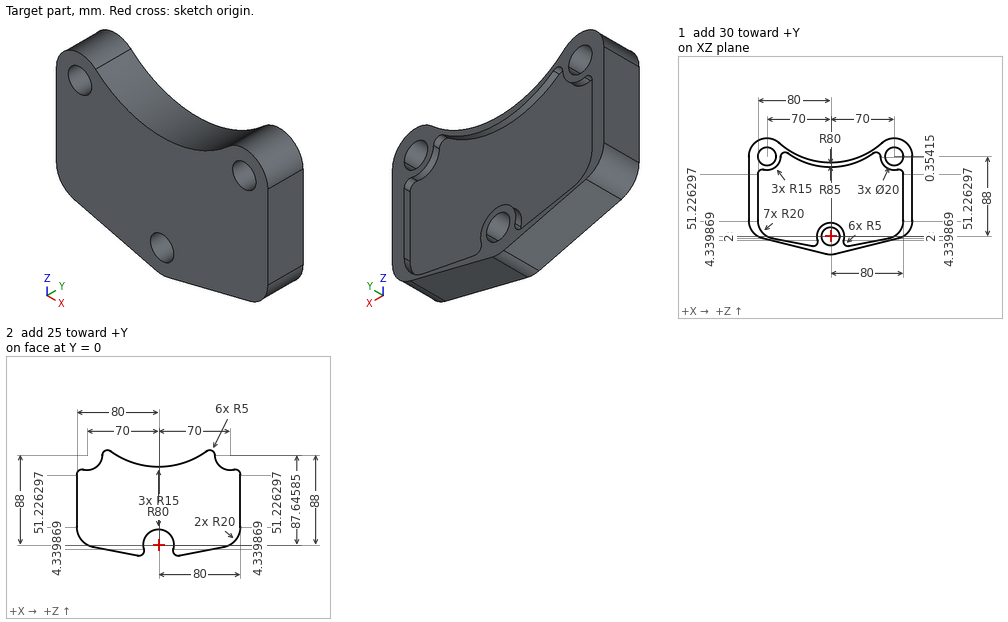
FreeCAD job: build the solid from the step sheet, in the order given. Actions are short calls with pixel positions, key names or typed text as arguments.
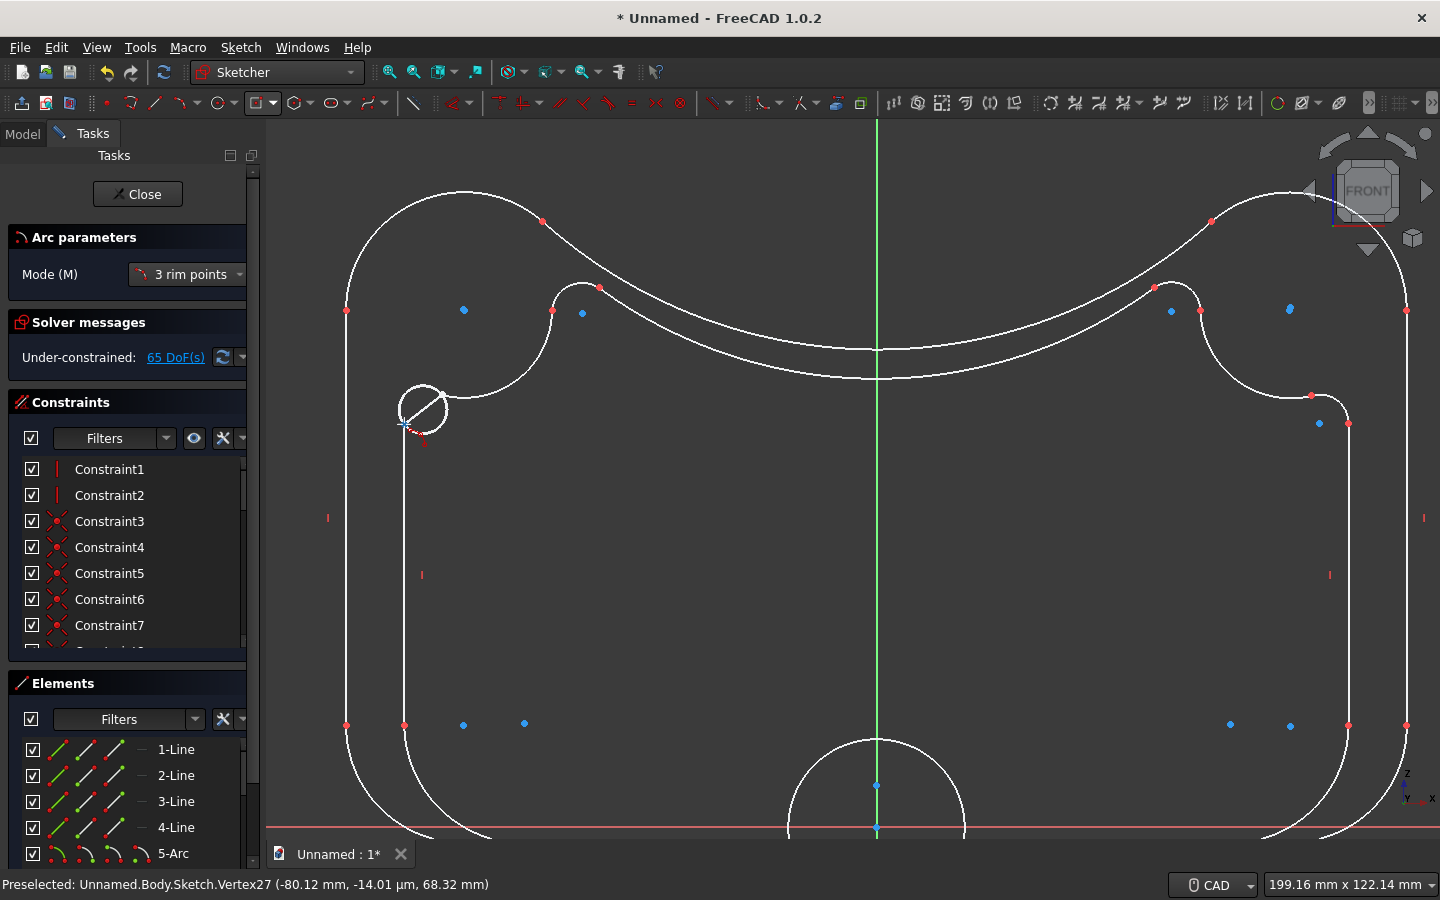
scroll(416, 399, up, 2)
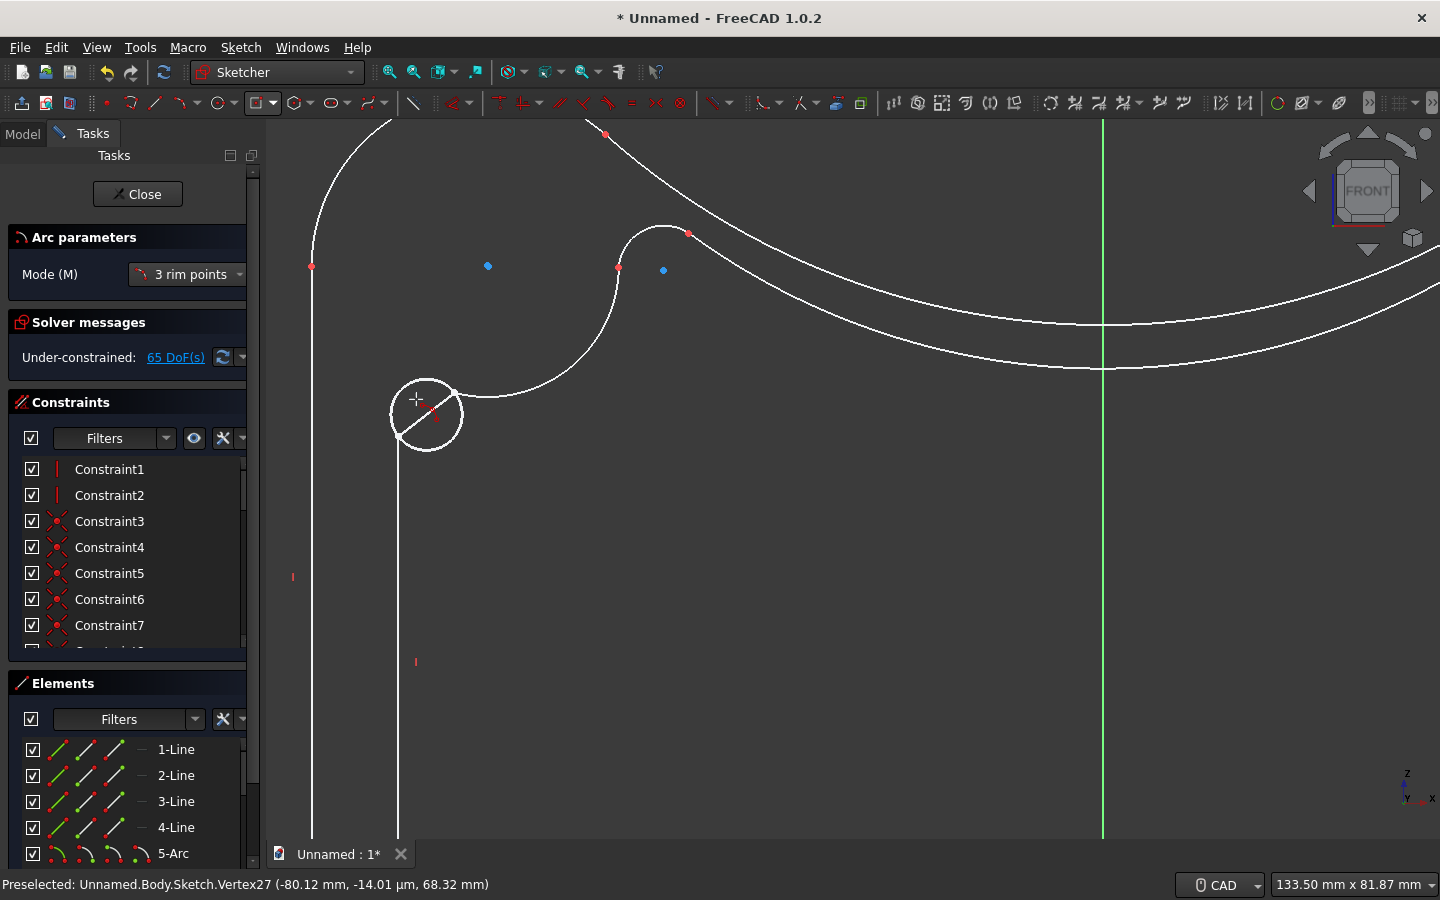
click(417, 399)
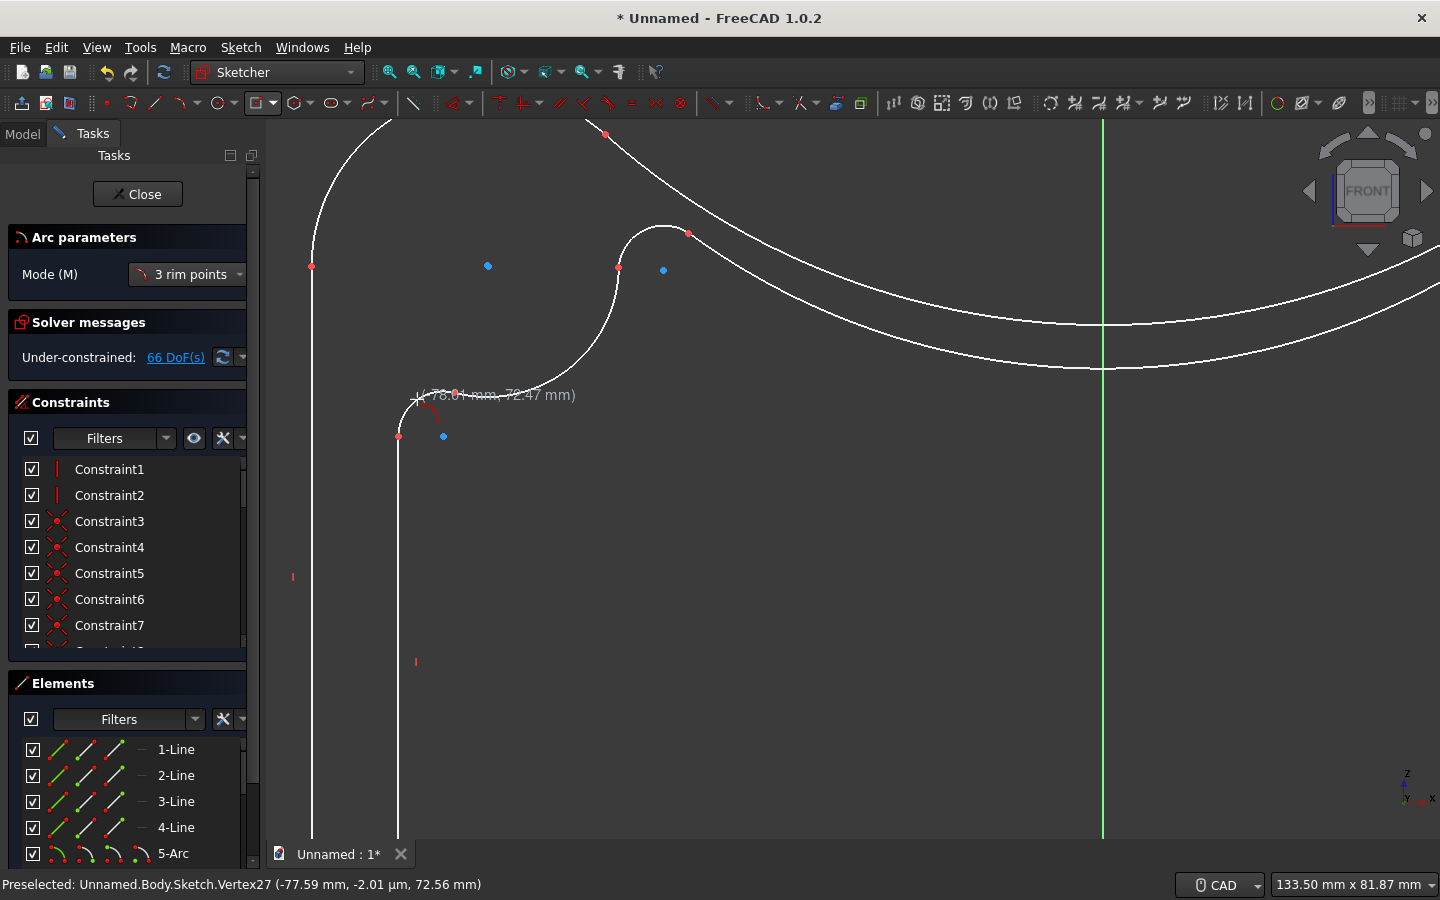
key(g)
key(c)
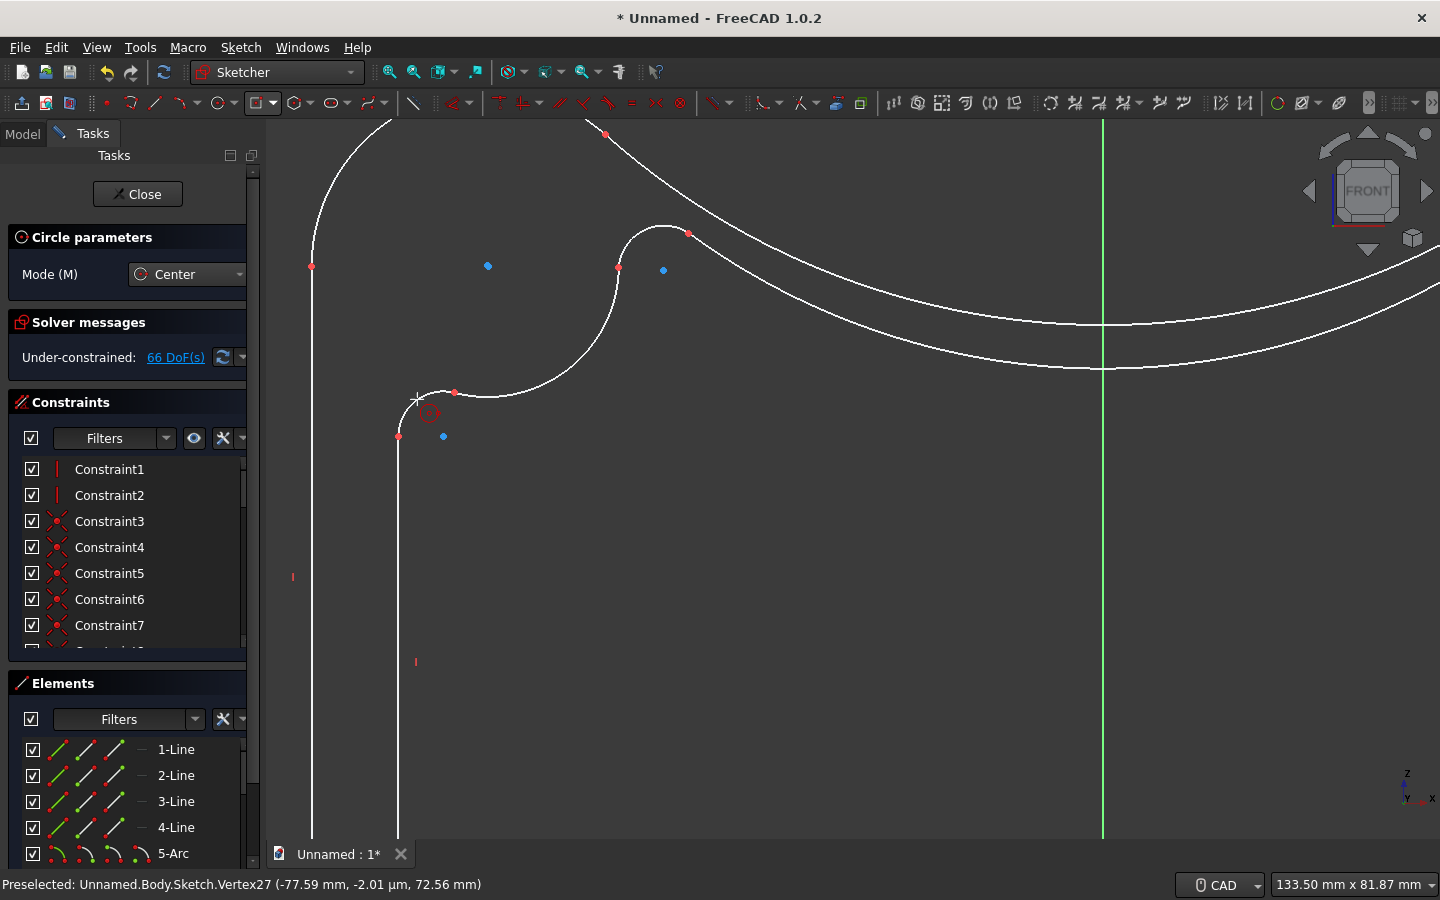
scroll(525, 333, down, 4)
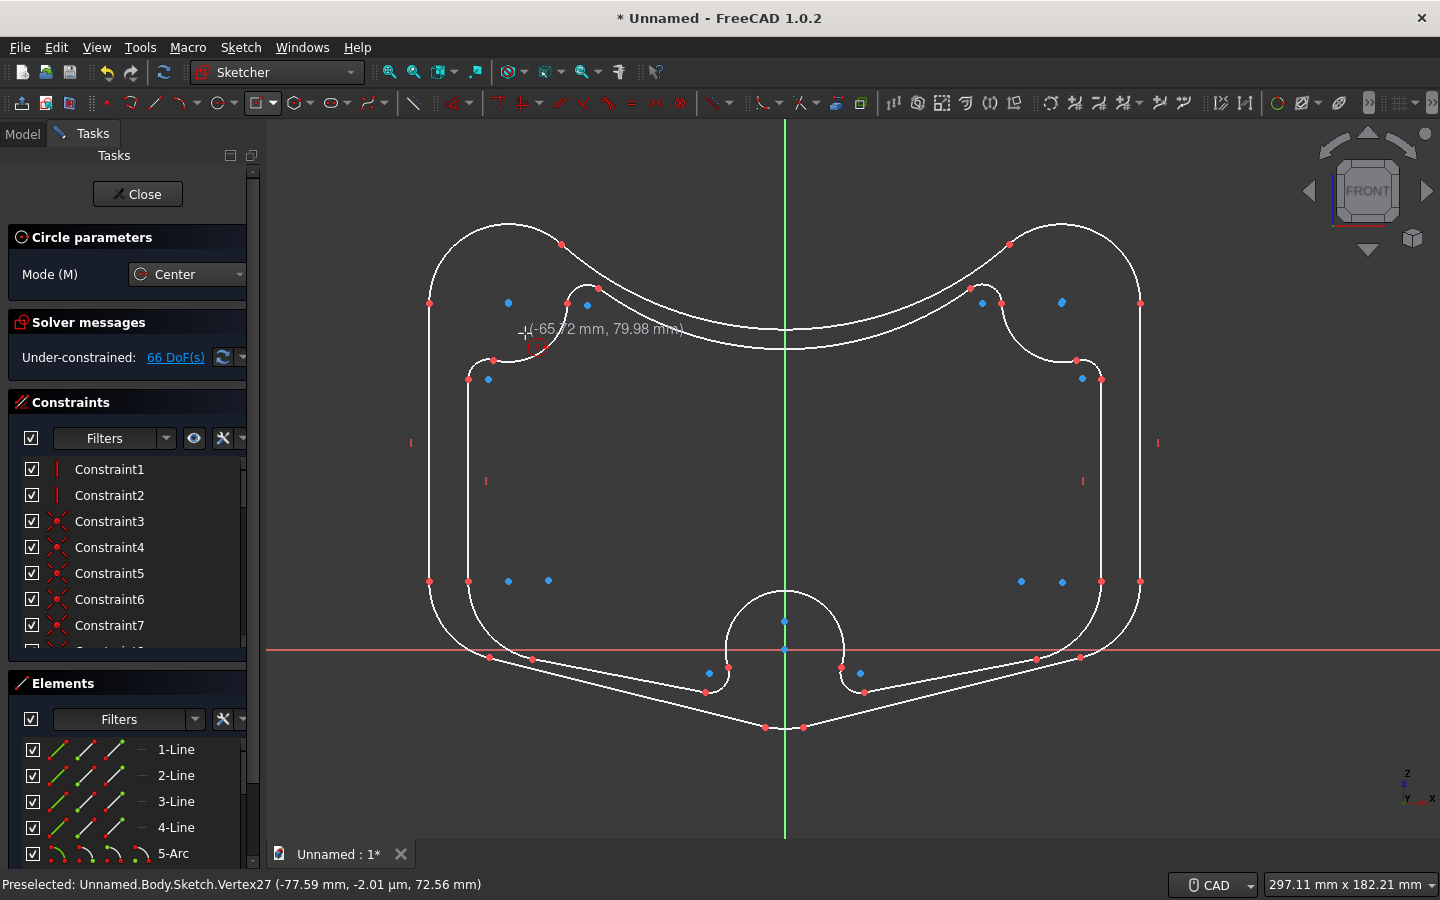
click(1061, 302)
move(1089, 274)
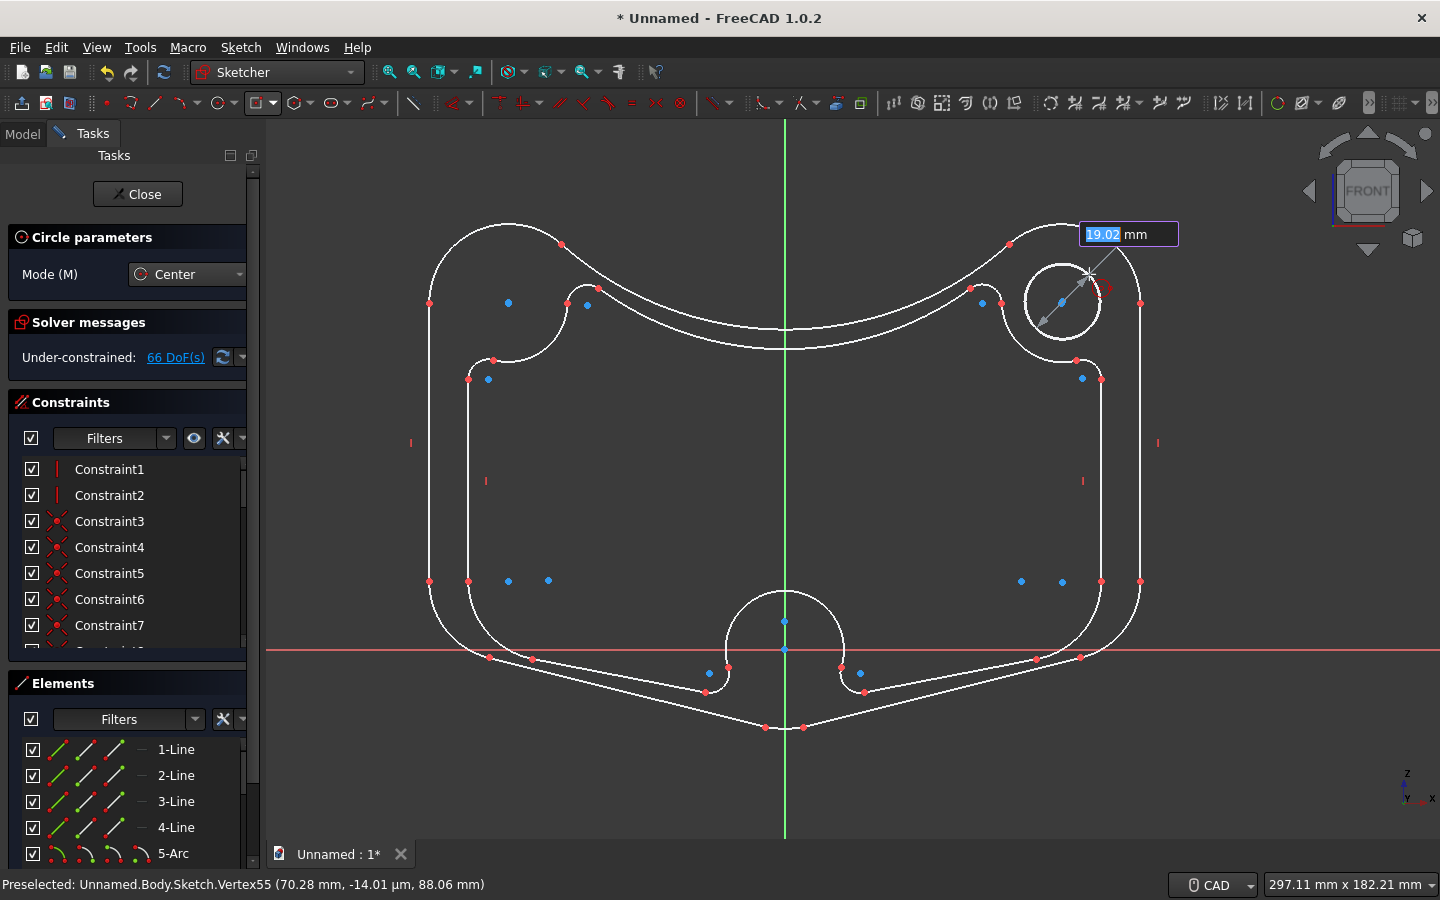
text(20)
key(Return)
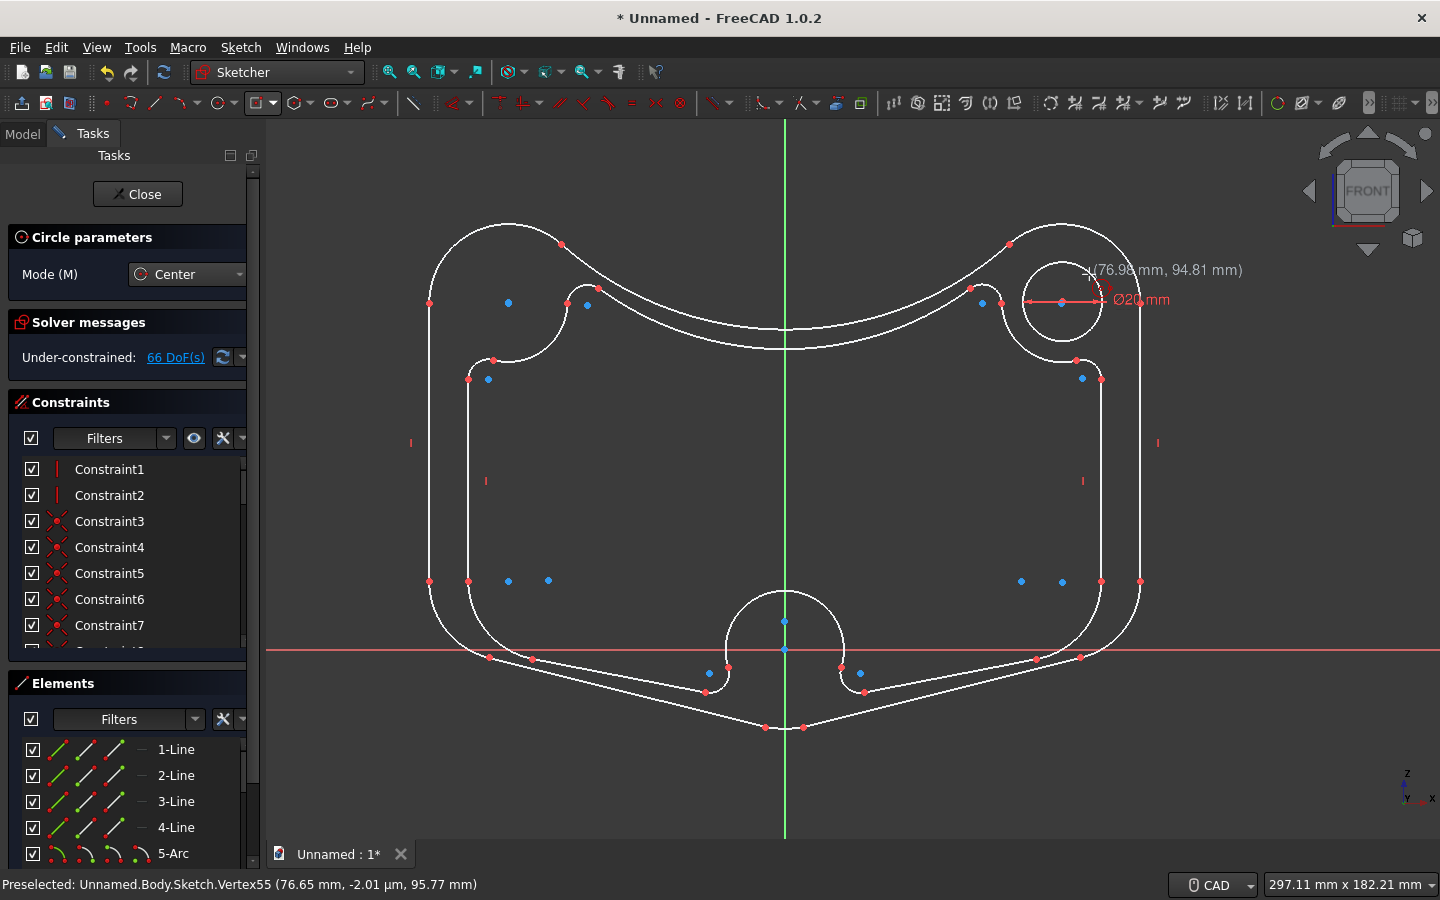
click(508, 302)
move(536, 274)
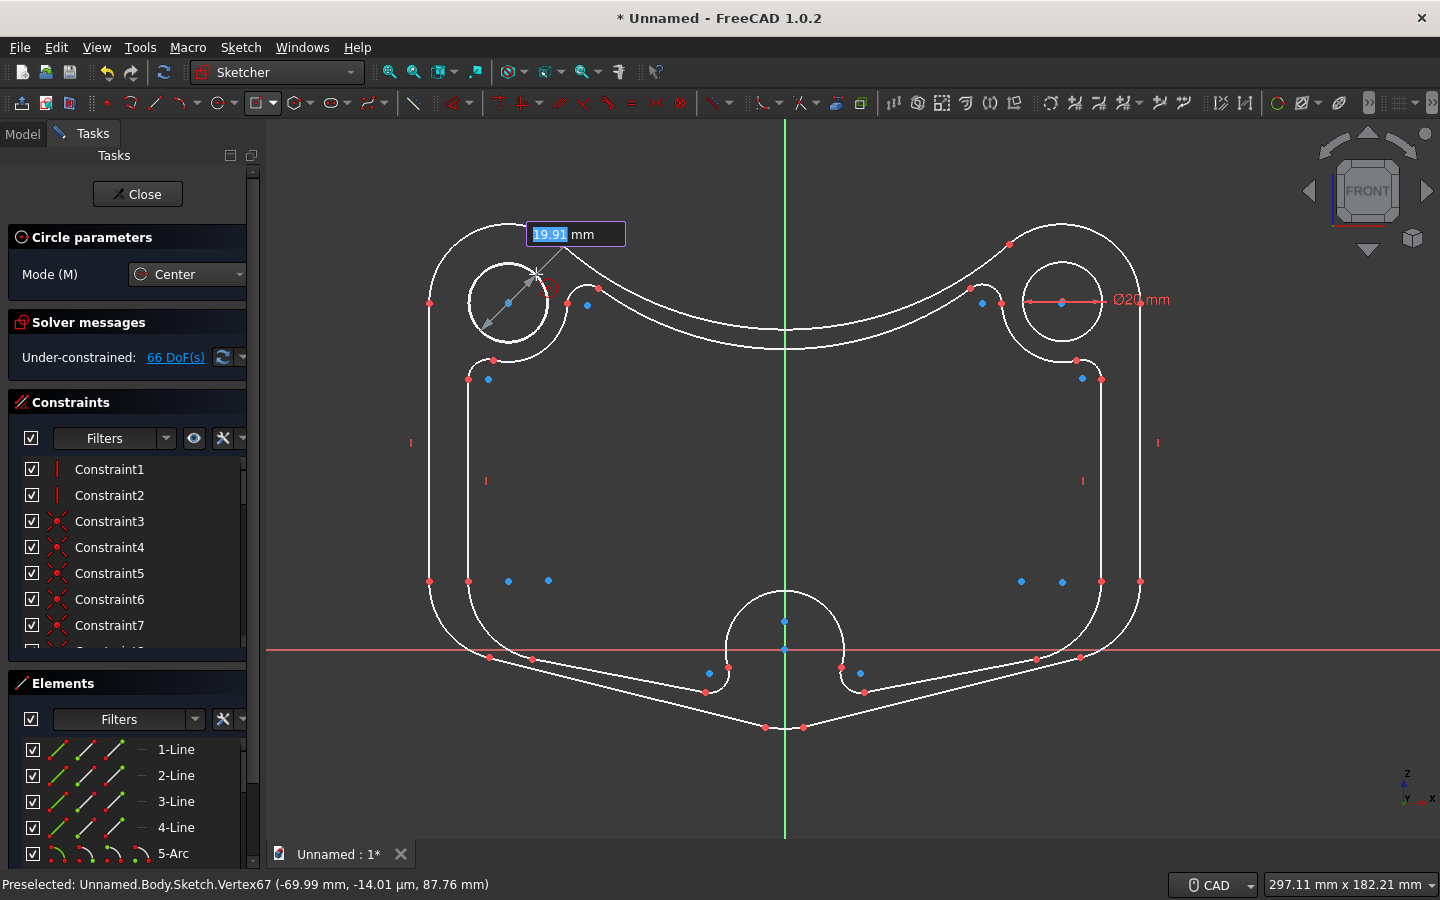
text(20)
key(Return)